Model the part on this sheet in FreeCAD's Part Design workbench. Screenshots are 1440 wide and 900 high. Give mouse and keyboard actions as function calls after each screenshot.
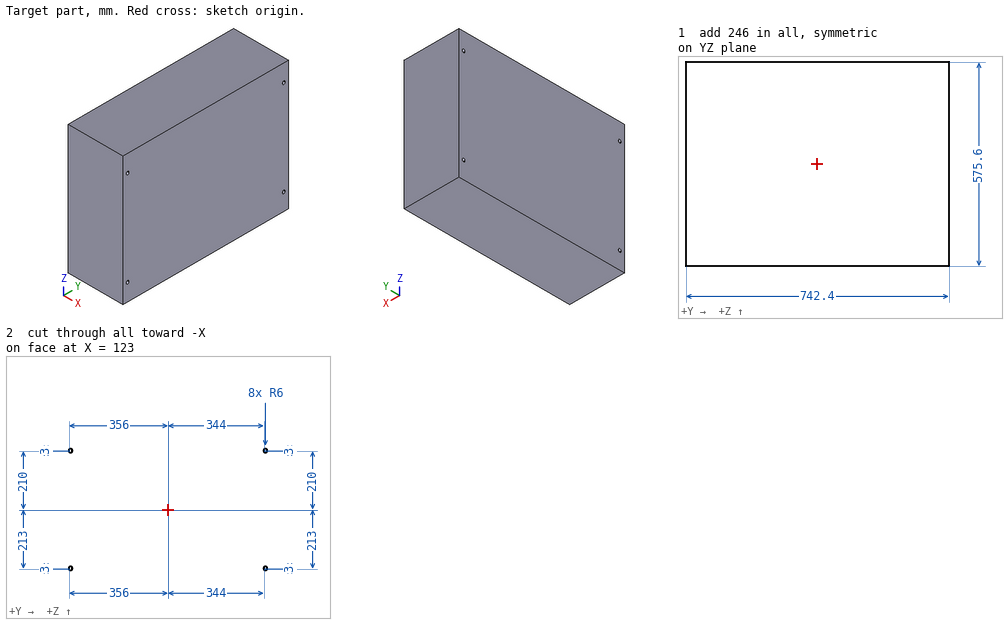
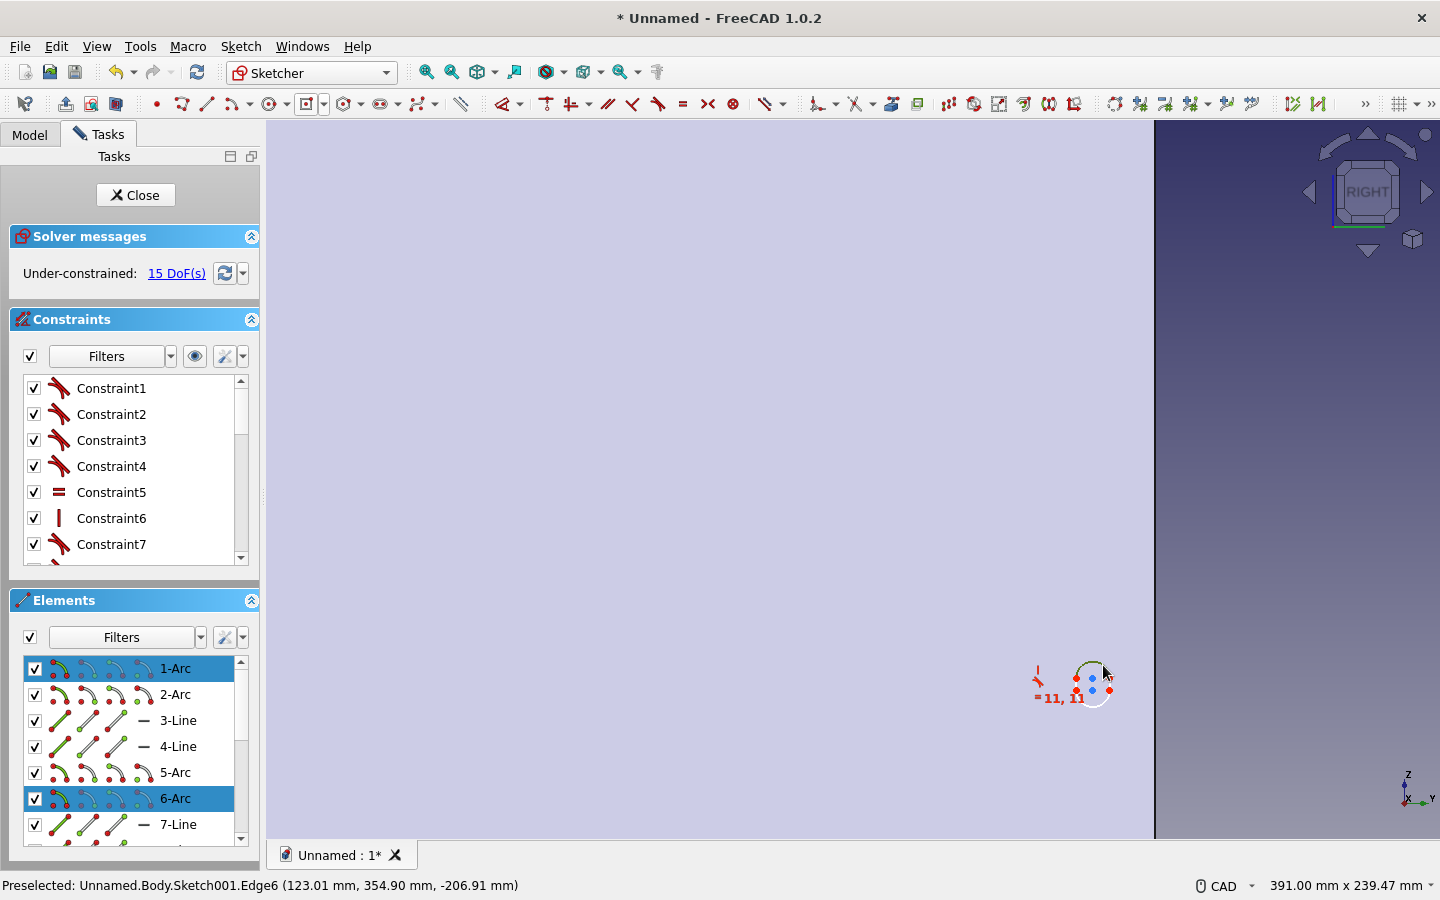
scroll(1105, 666, down, 6)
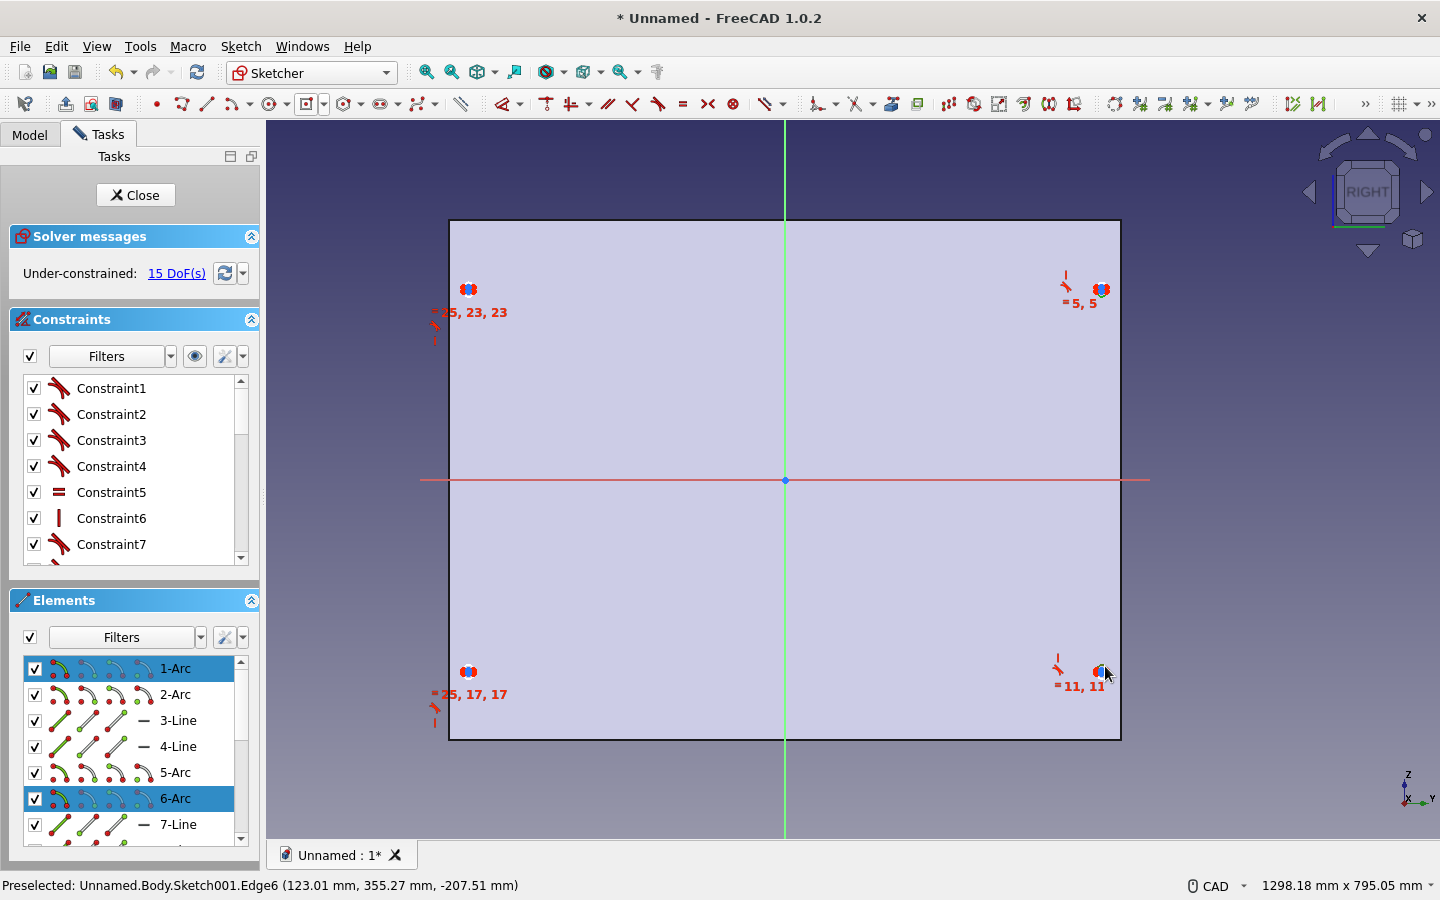
scroll(472, 666, up, 6)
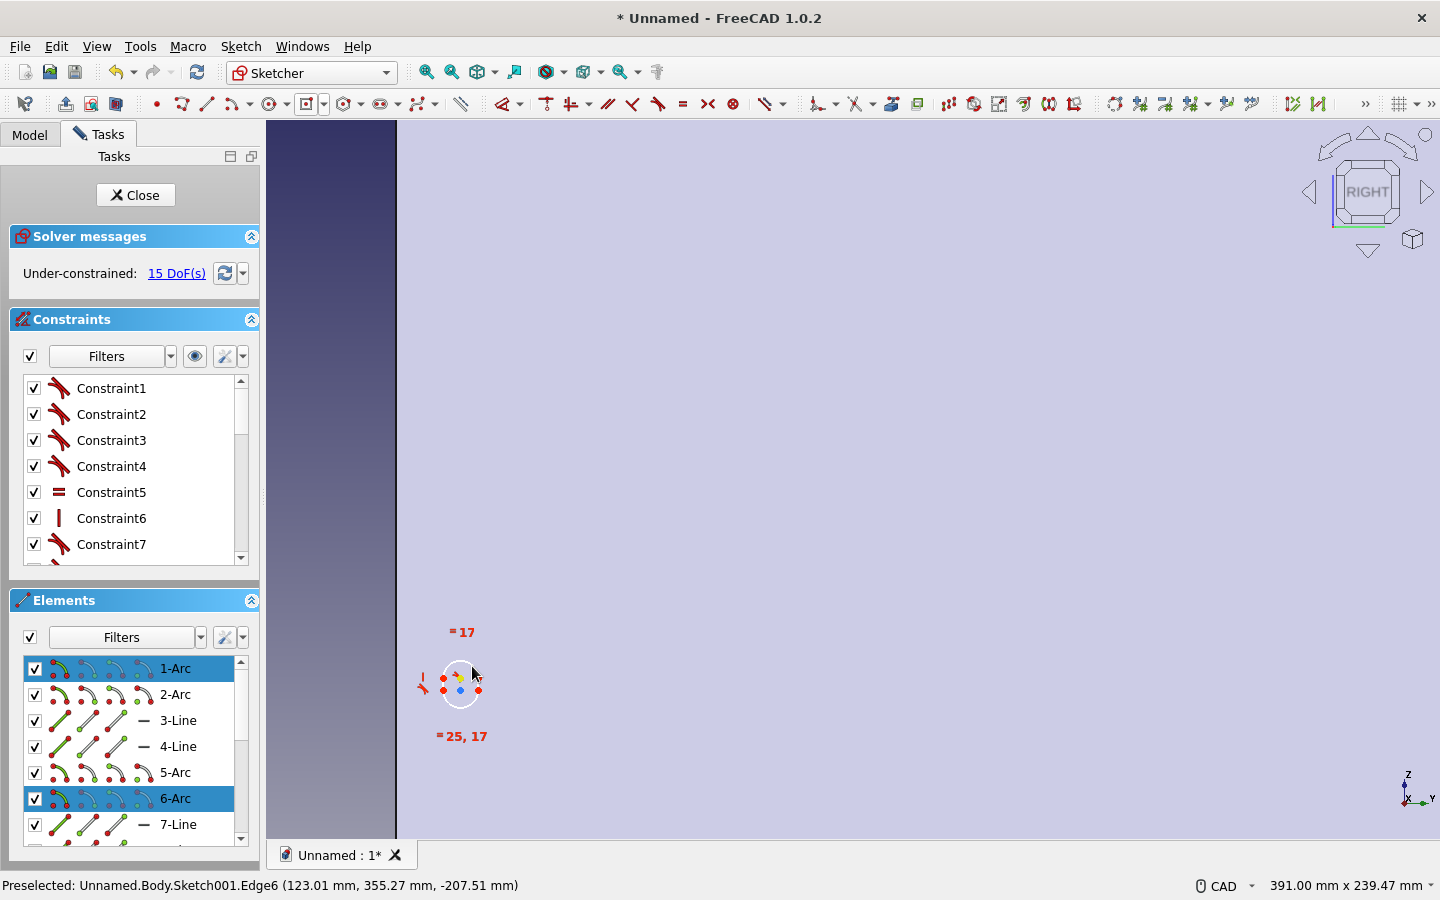
click(471, 664)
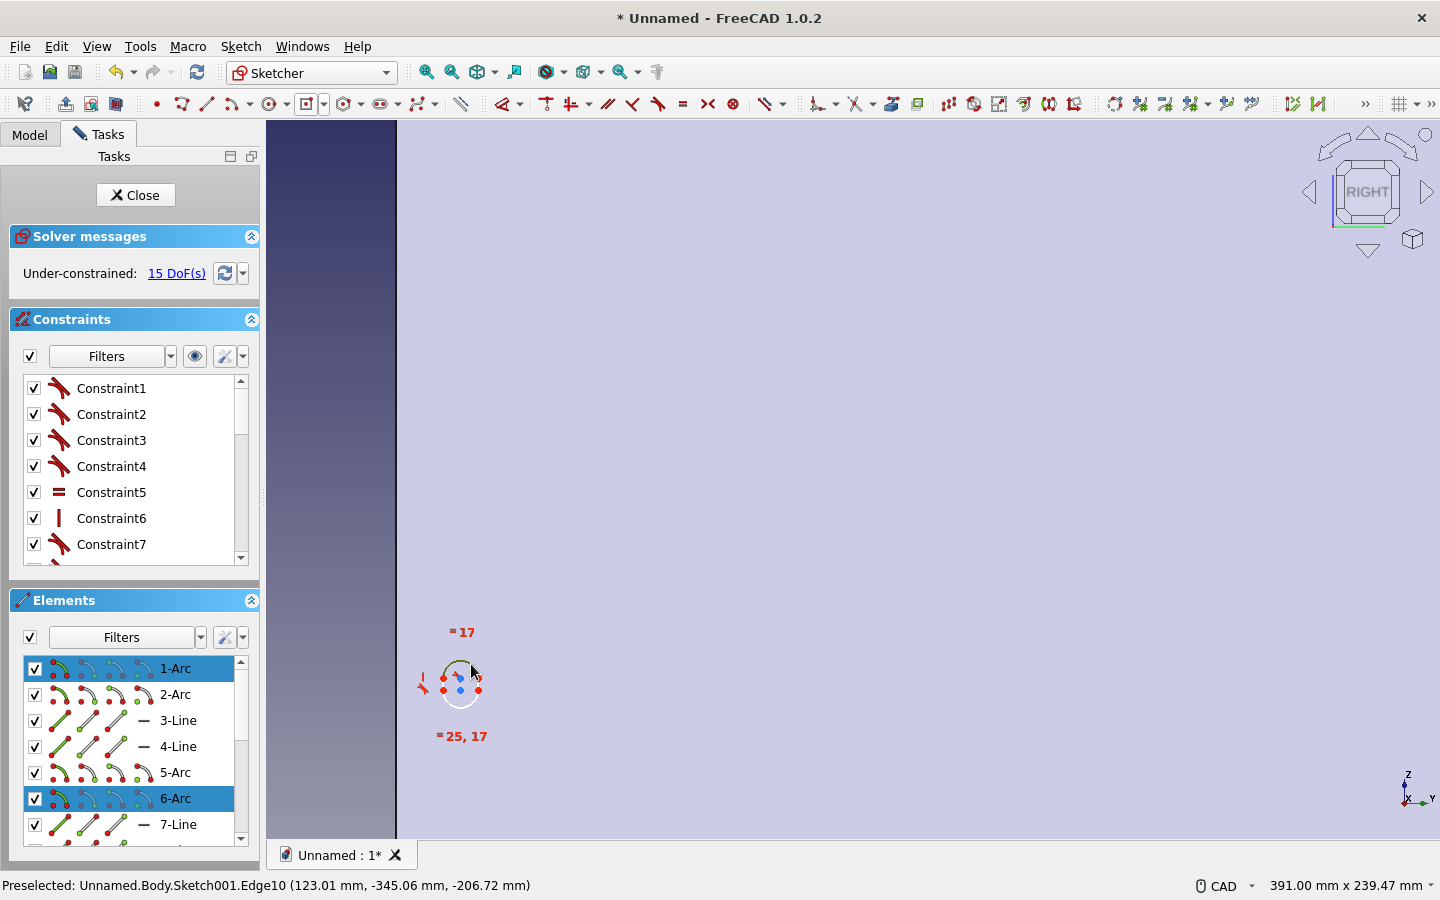
key(e)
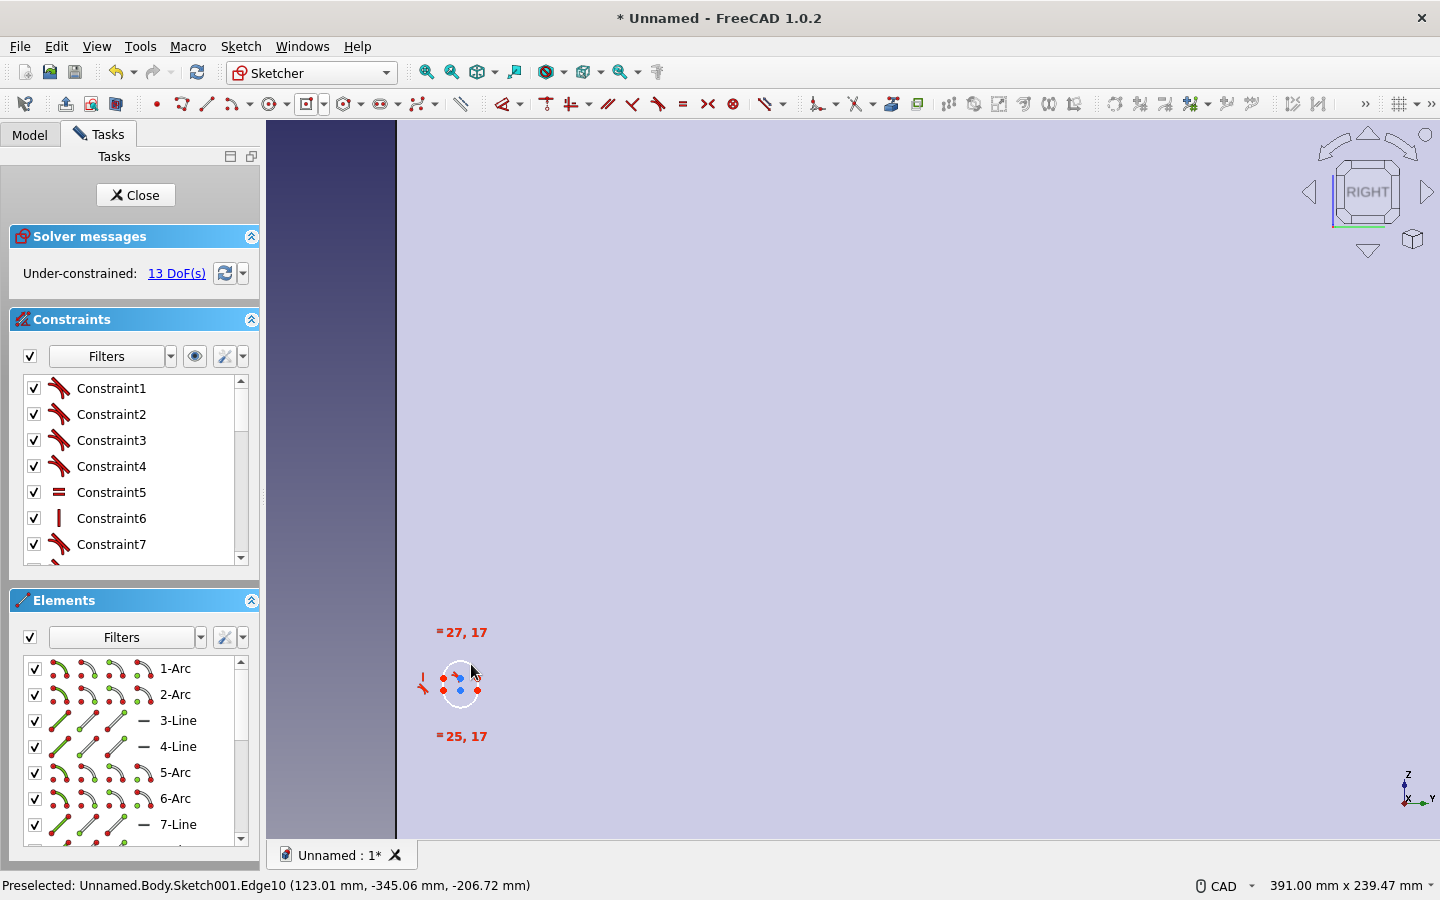
click(502, 104)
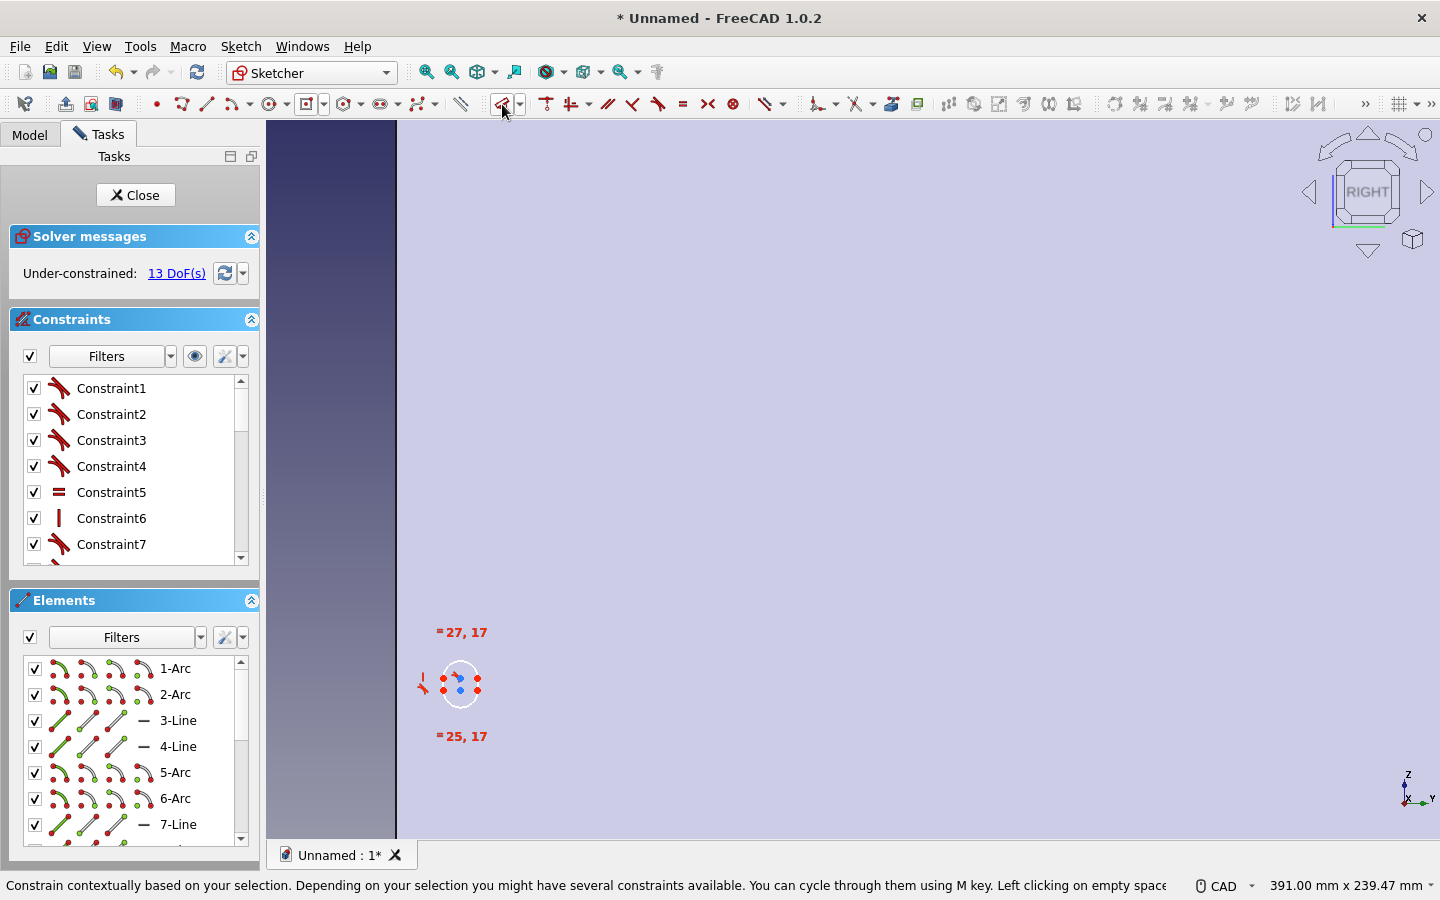
scroll(471, 666, down, 6)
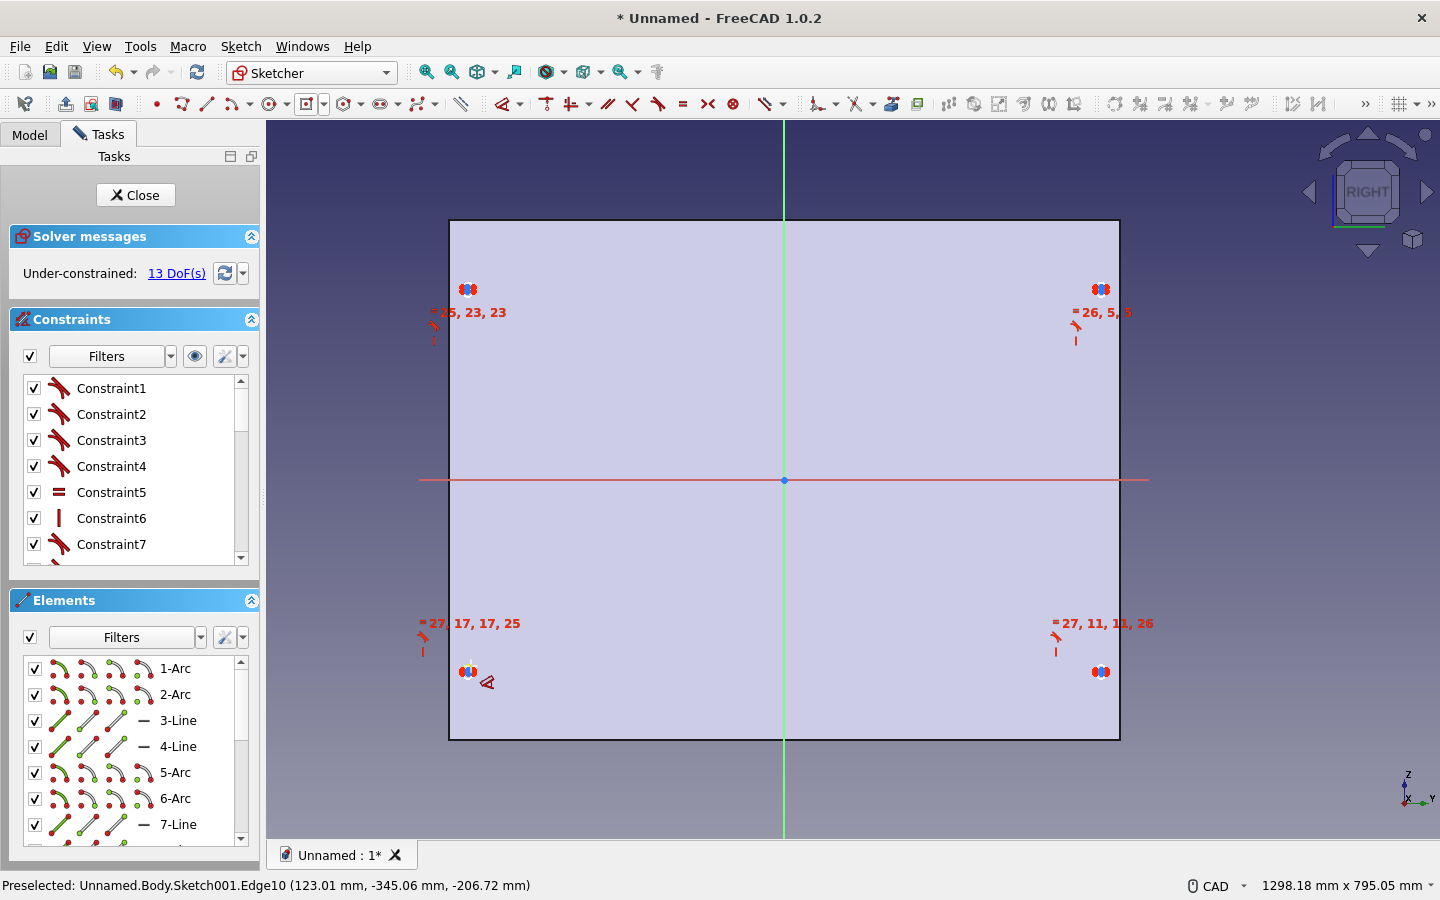
scroll(1098, 296, up, 10)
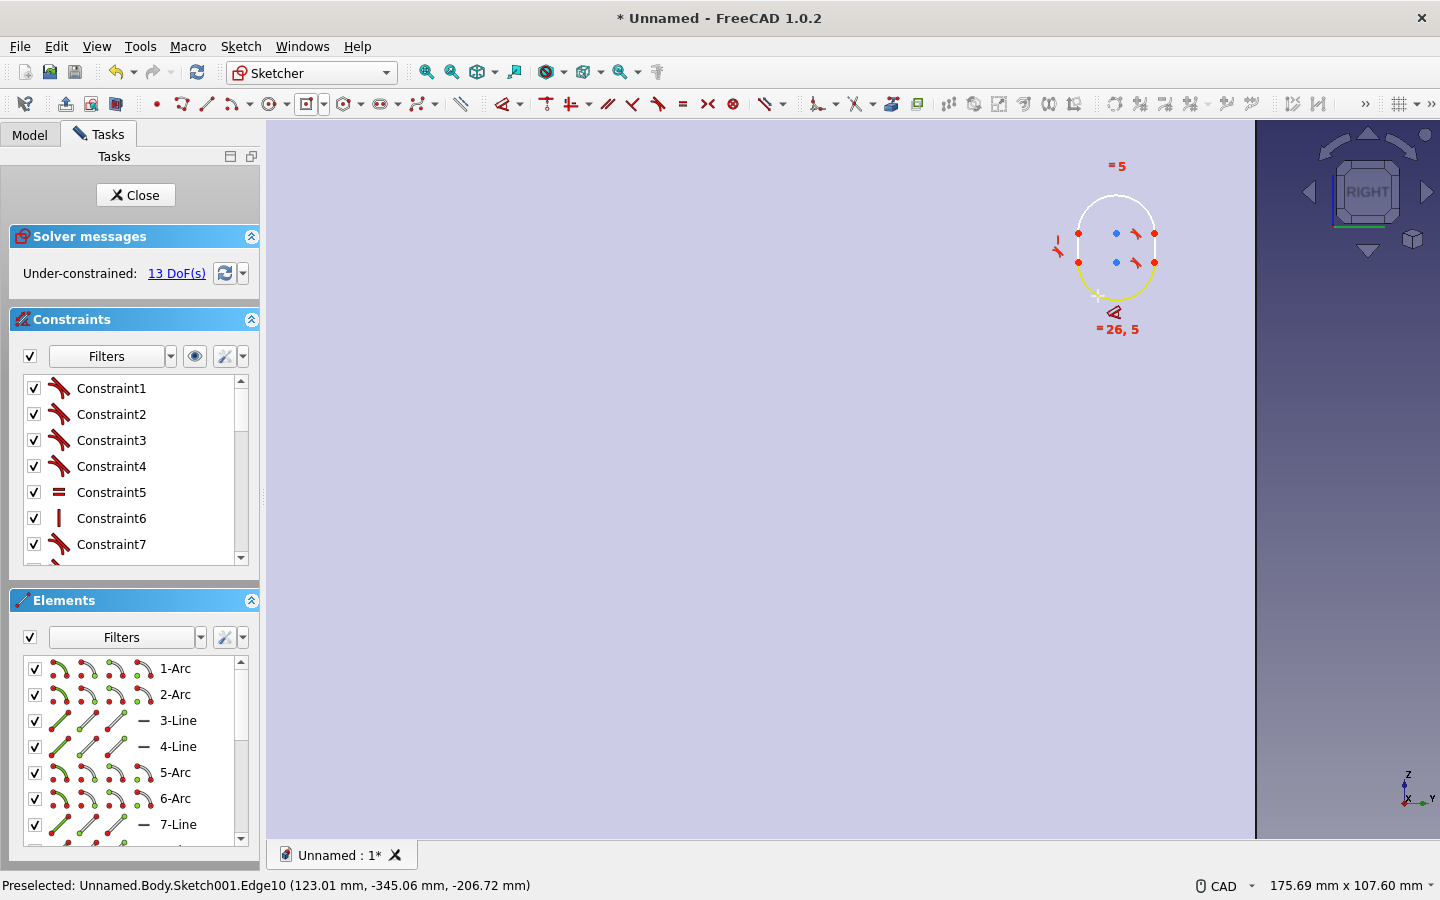
click(1094, 293)
click(1075, 319)